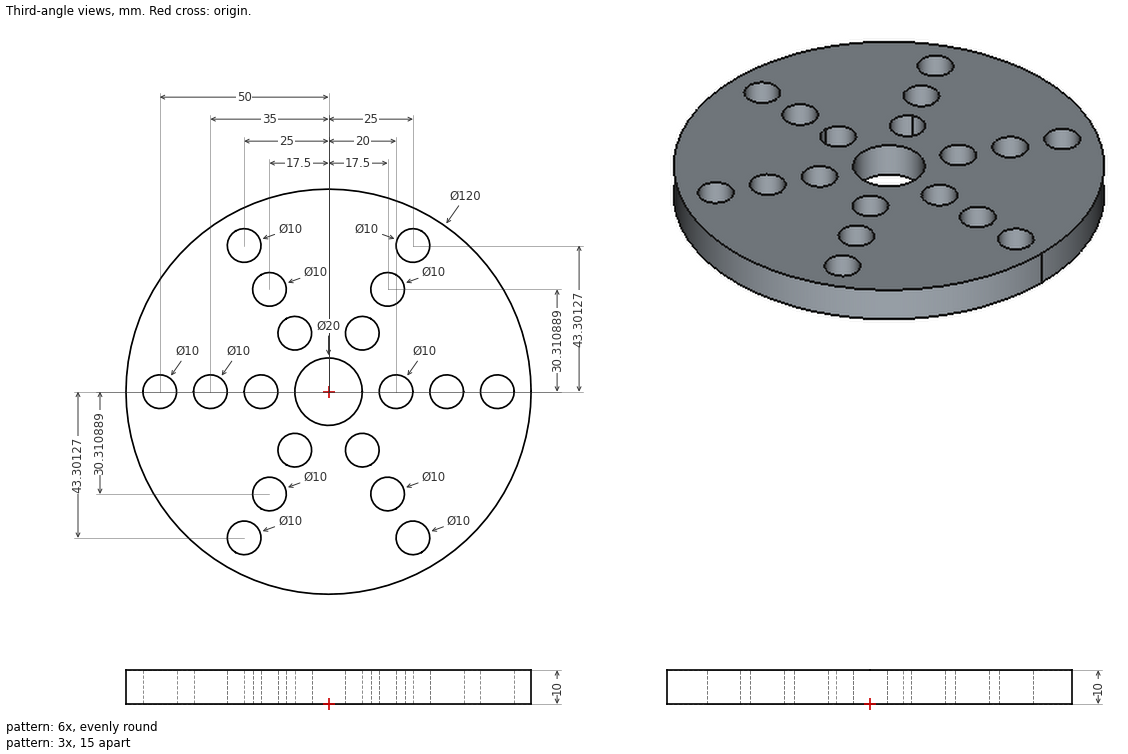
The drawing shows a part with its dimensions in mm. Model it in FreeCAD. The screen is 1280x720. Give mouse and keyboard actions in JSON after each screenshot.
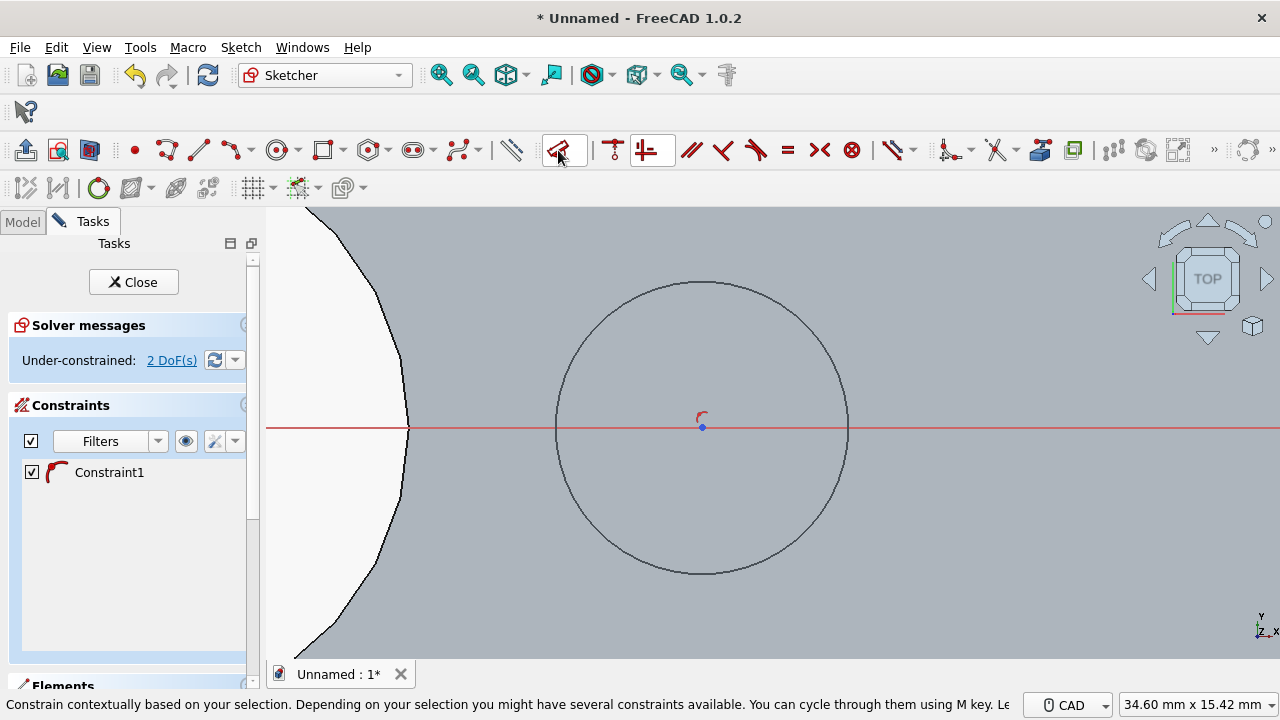
{"action": "left_click", "coordinate": [805, 324]}
{"action": "left_click", "coordinate": [828, 301]}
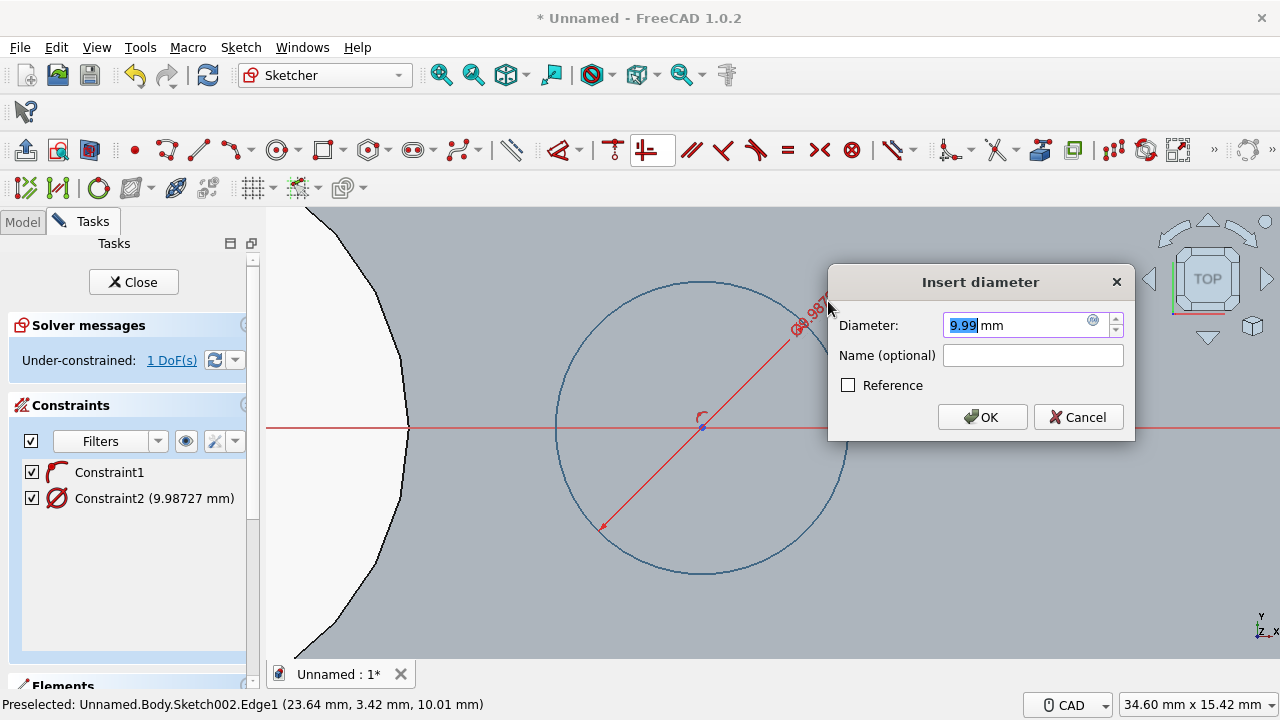
{"action": "type", "text": "10"}
{"action": "key", "text": "Return"}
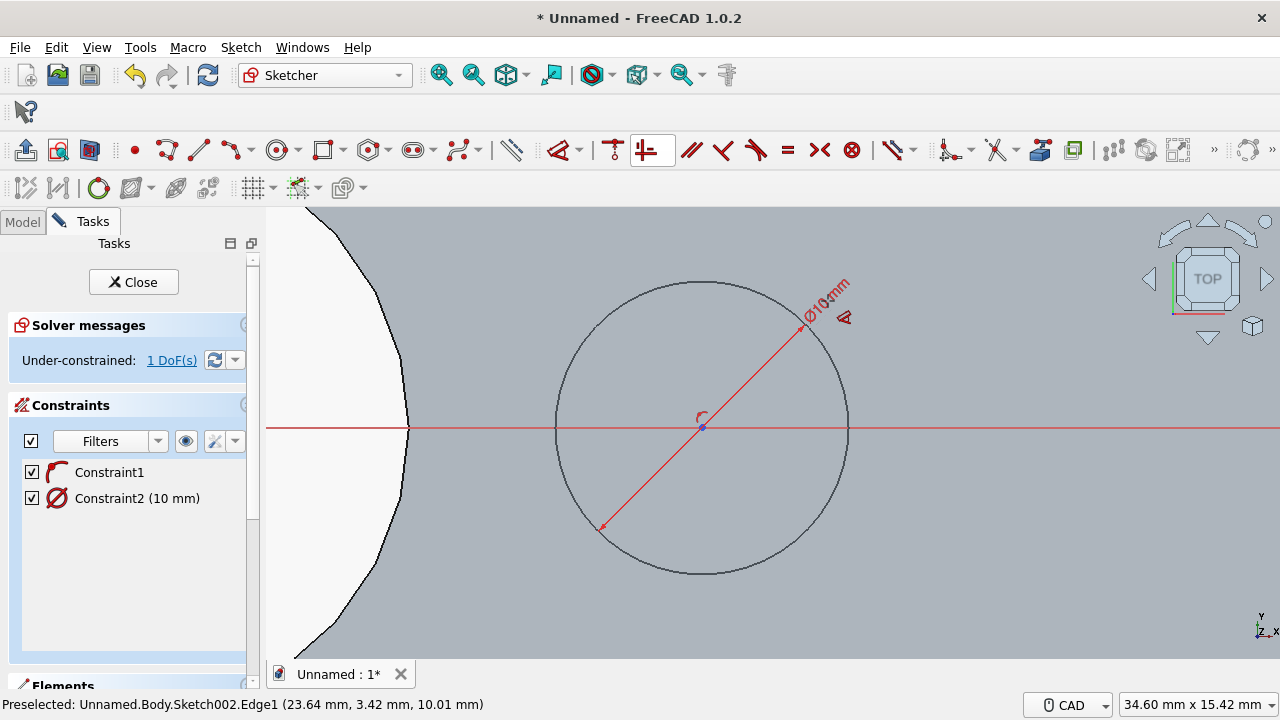
{"action": "left_click", "coordinate": [702, 428]}
{"action": "left_click", "coordinate": [498, 462]}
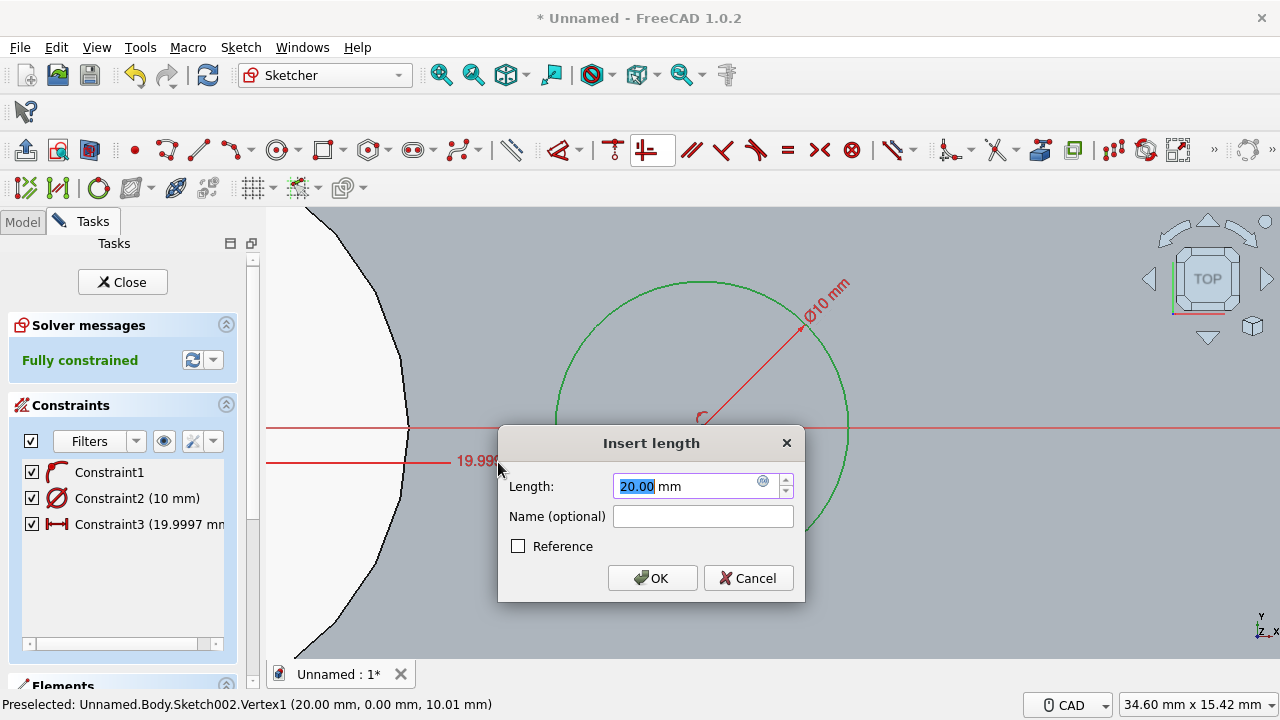
{"action": "type", "text": "20"}
{"action": "key", "text": "Return"}
{"action": "key", "text": "Escape"}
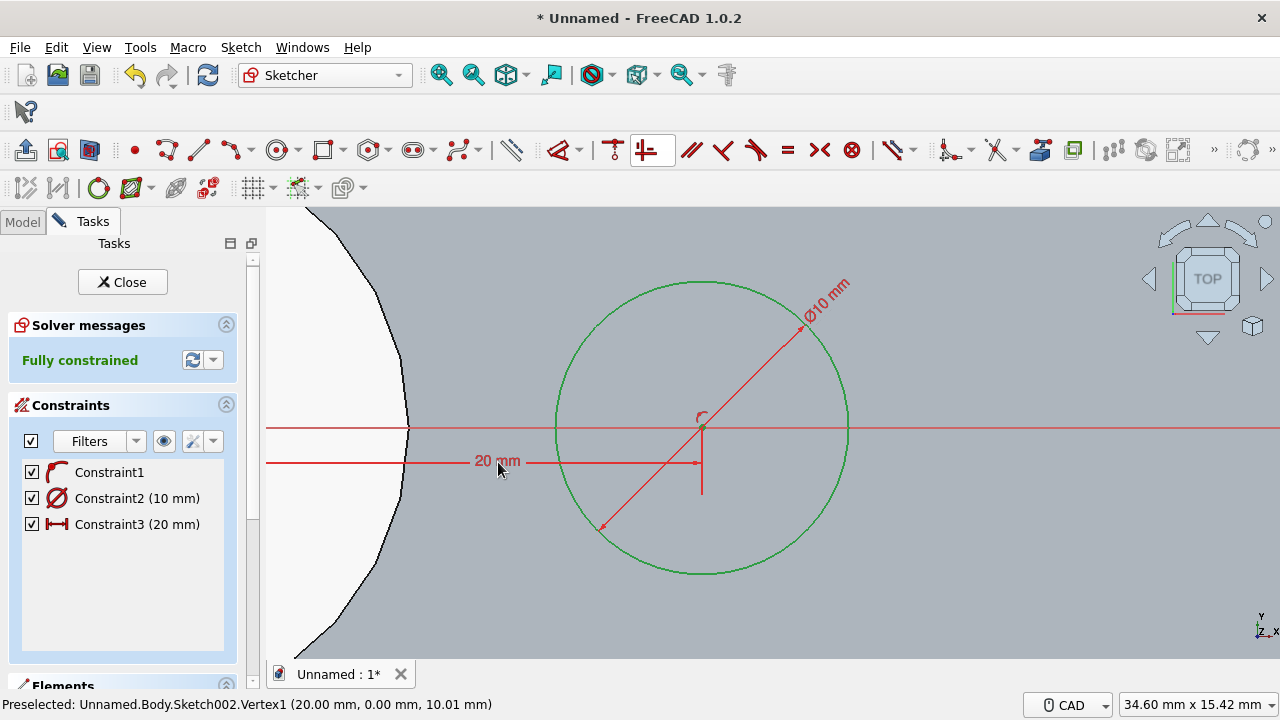
{"action": "left_click", "coordinate": [123, 282]}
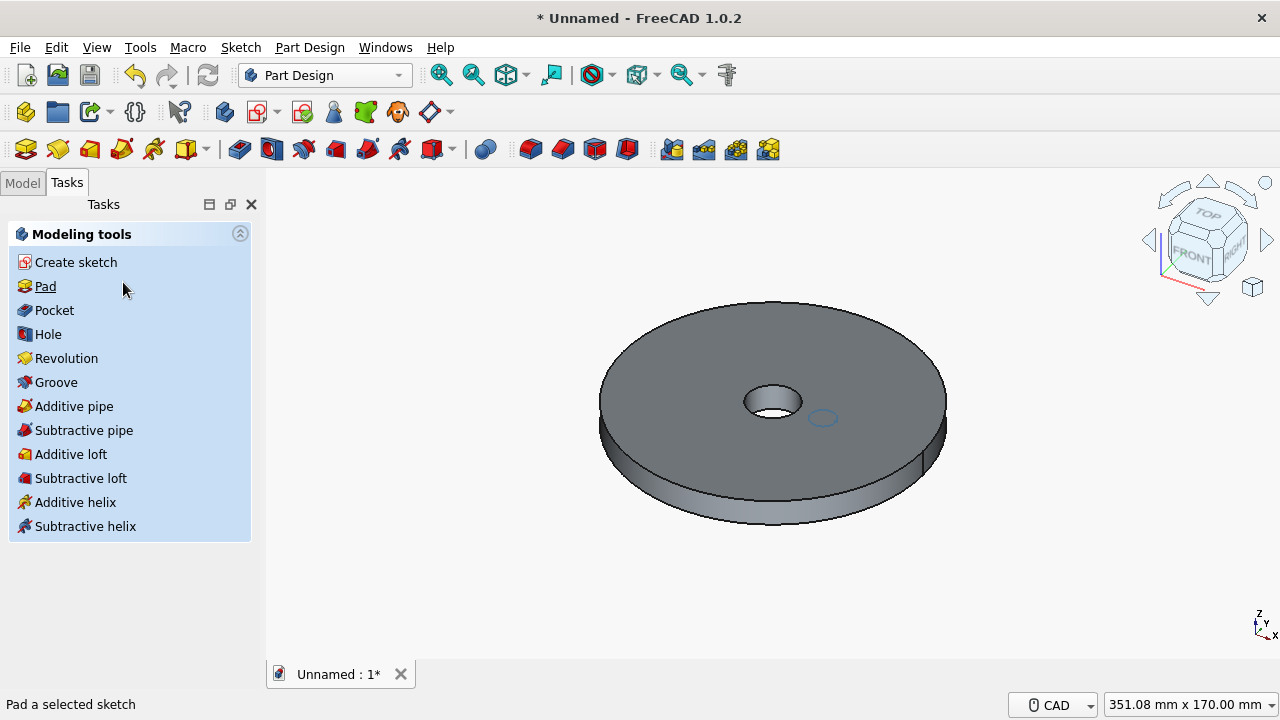
{"action": "left_click", "coordinate": [240, 150]}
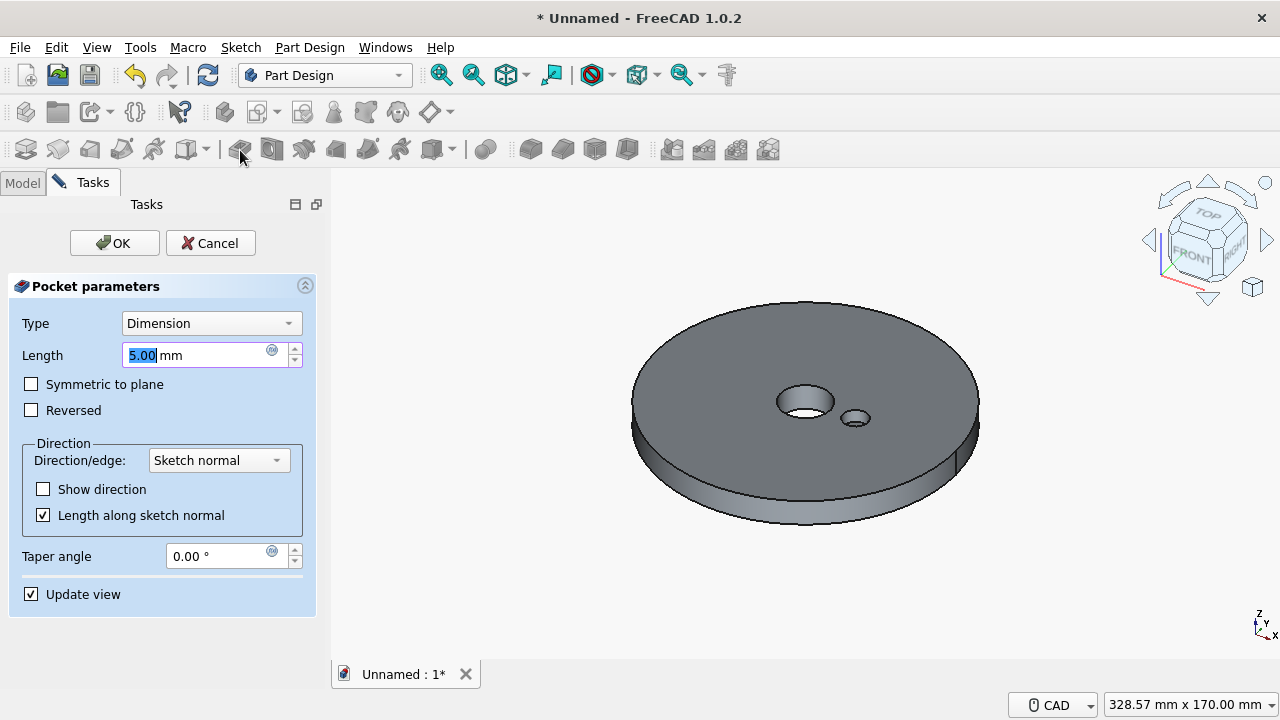
{"action": "type", "text": "10"}
{"action": "key", "text": "Tab"}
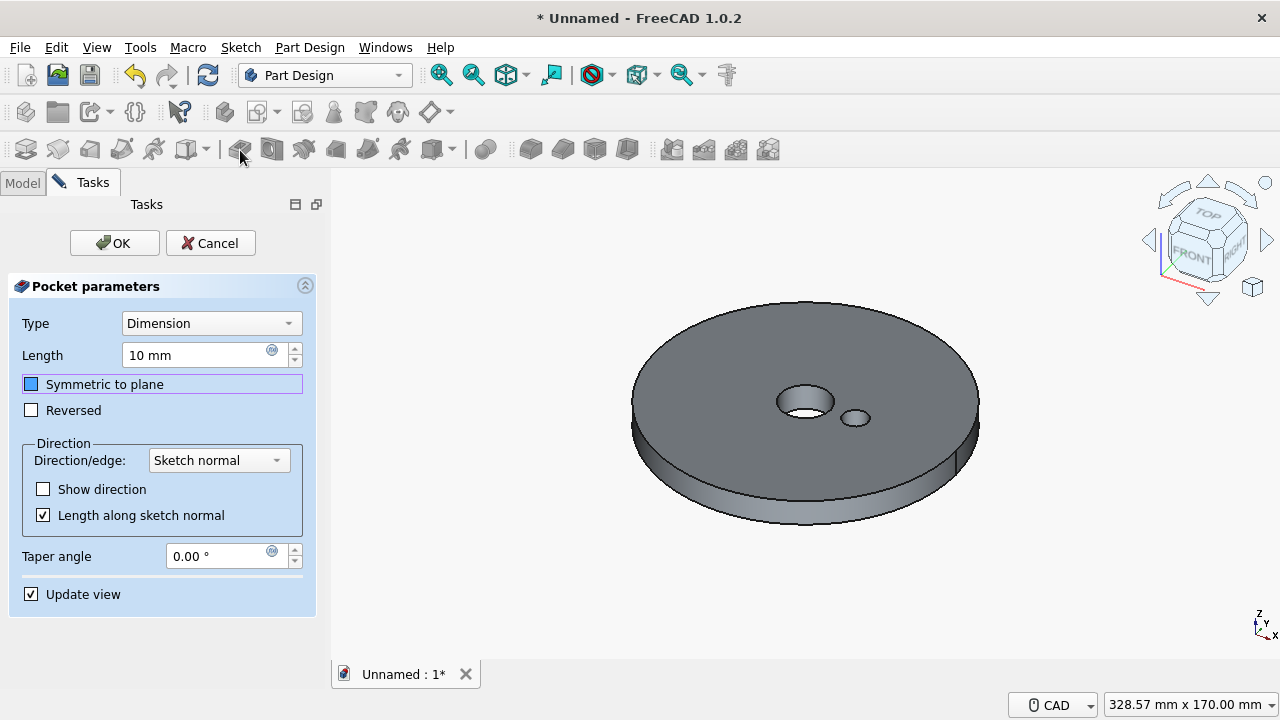
{"action": "left_click", "coordinate": [115, 243]}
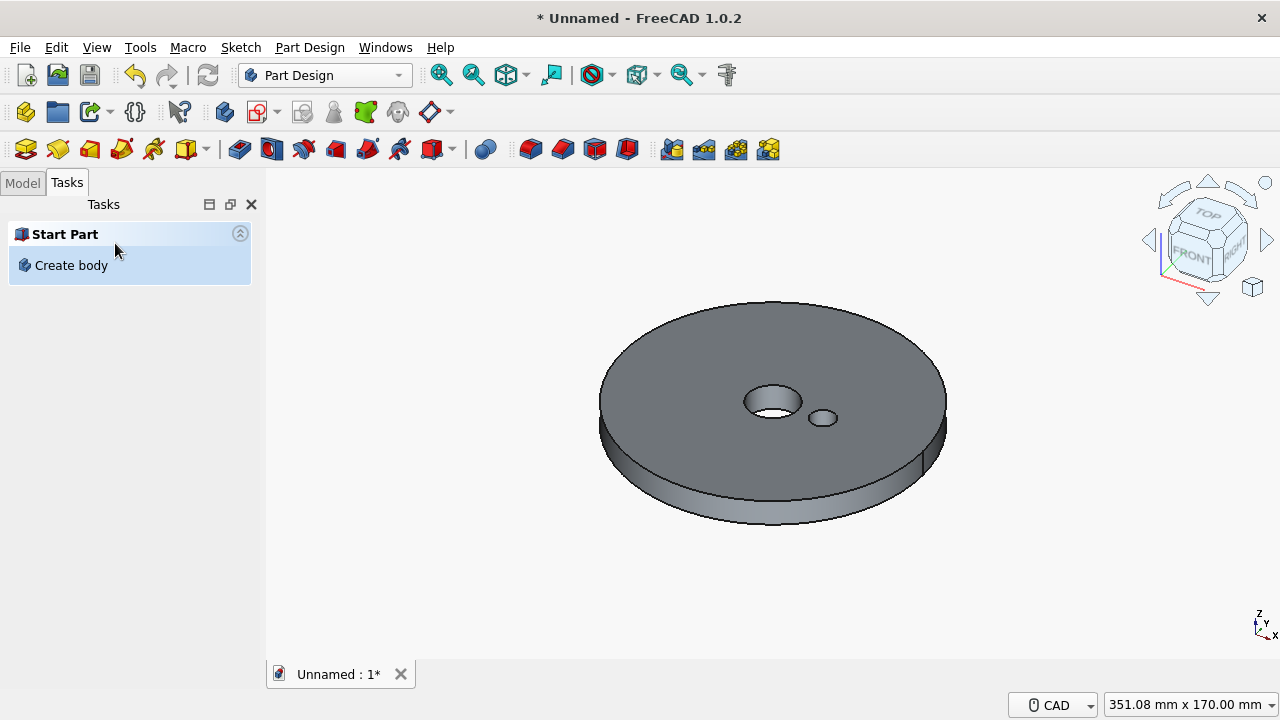
{"action": "left_click", "coordinate": [23, 182]}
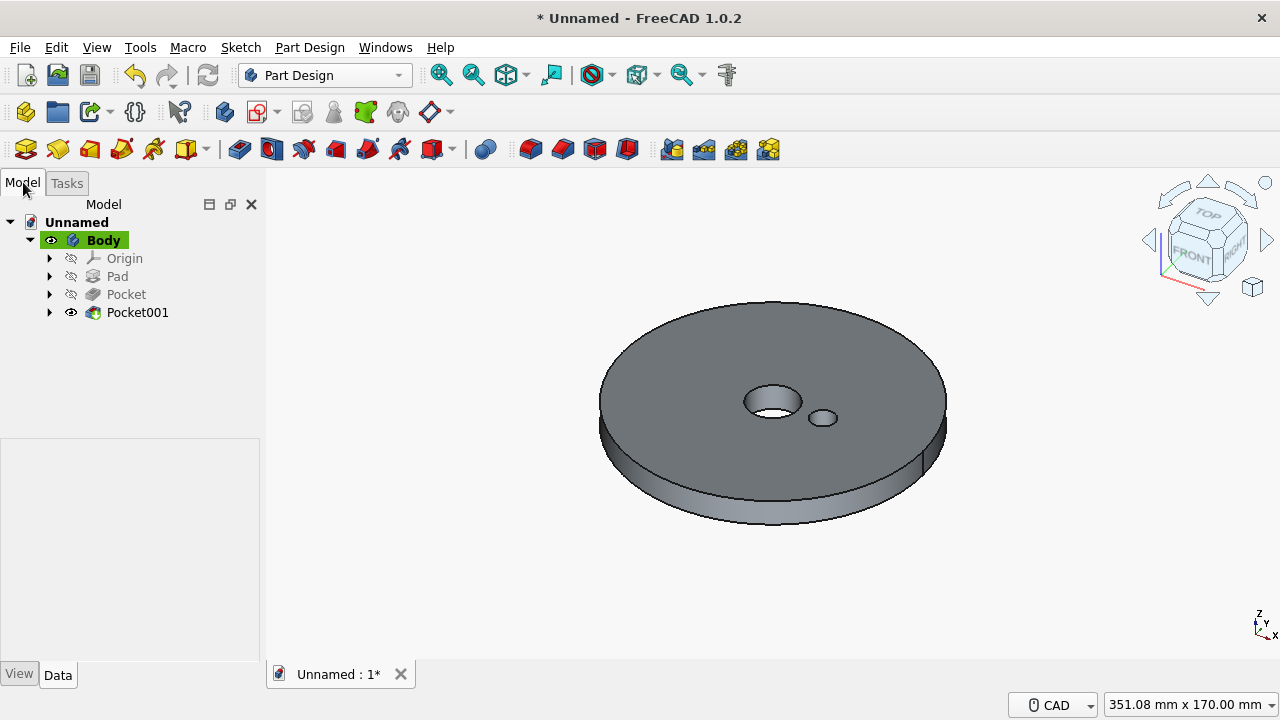
{"action": "left_click", "coordinate": [116, 312]}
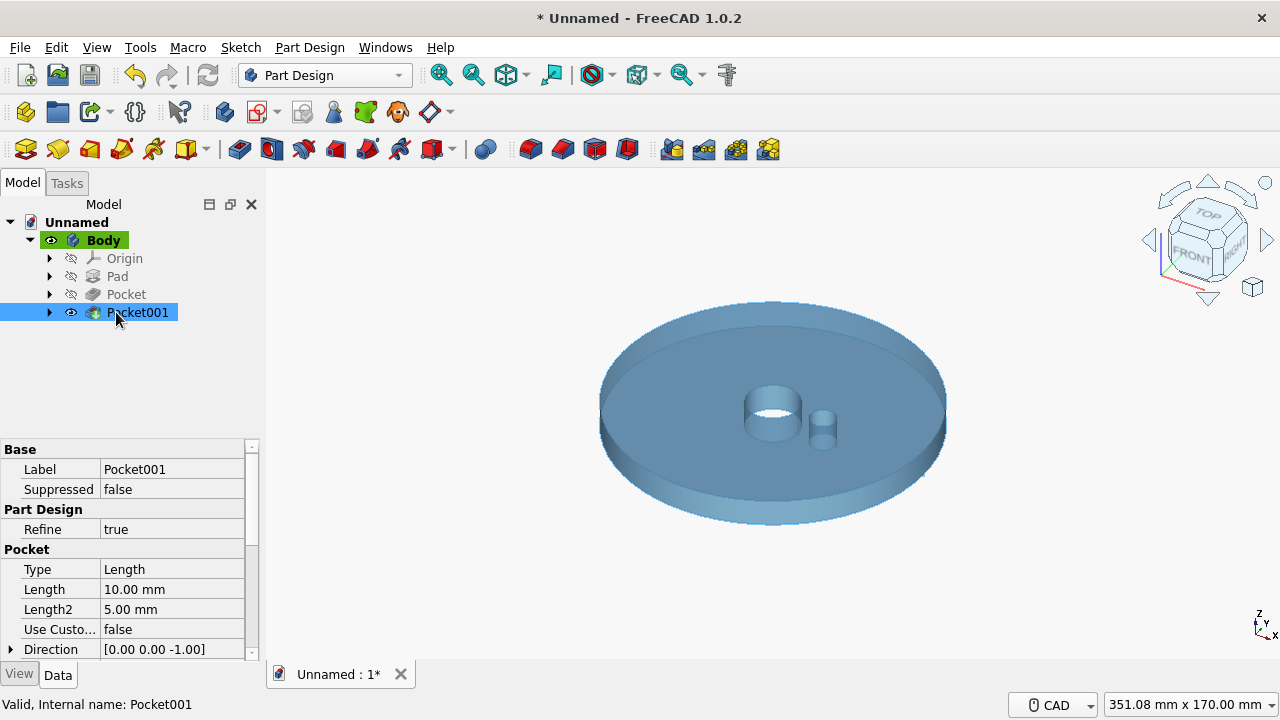
{"action": "left_click", "coordinate": [736, 150]}